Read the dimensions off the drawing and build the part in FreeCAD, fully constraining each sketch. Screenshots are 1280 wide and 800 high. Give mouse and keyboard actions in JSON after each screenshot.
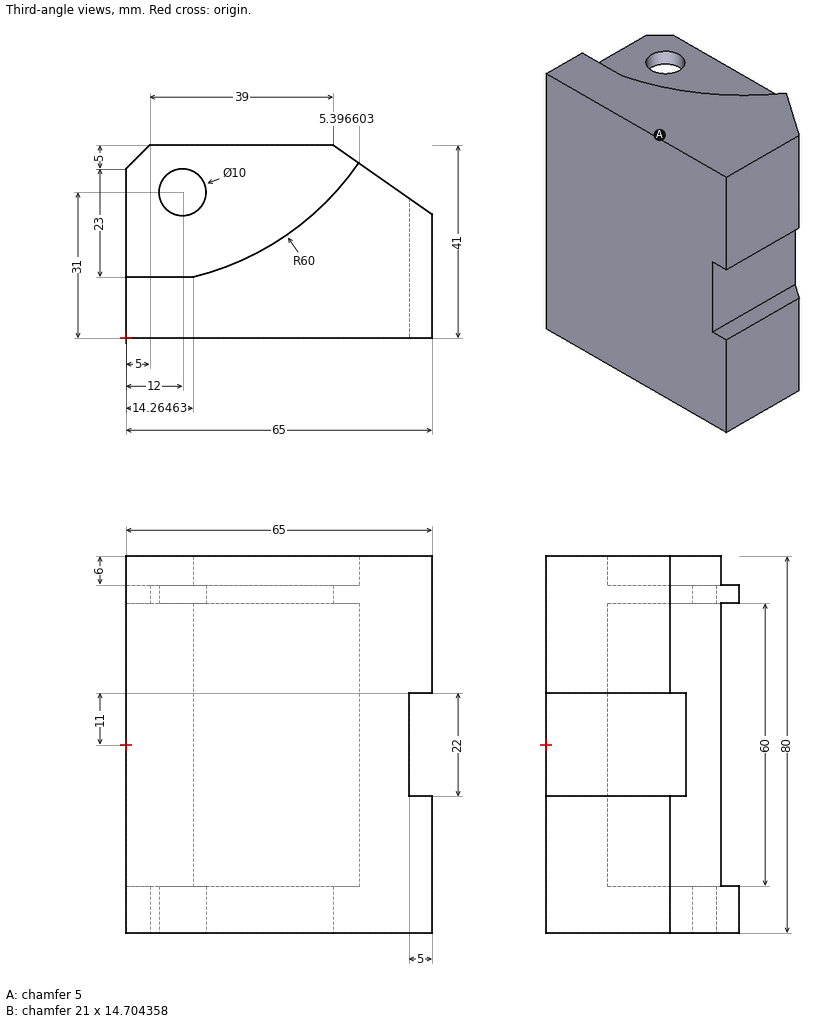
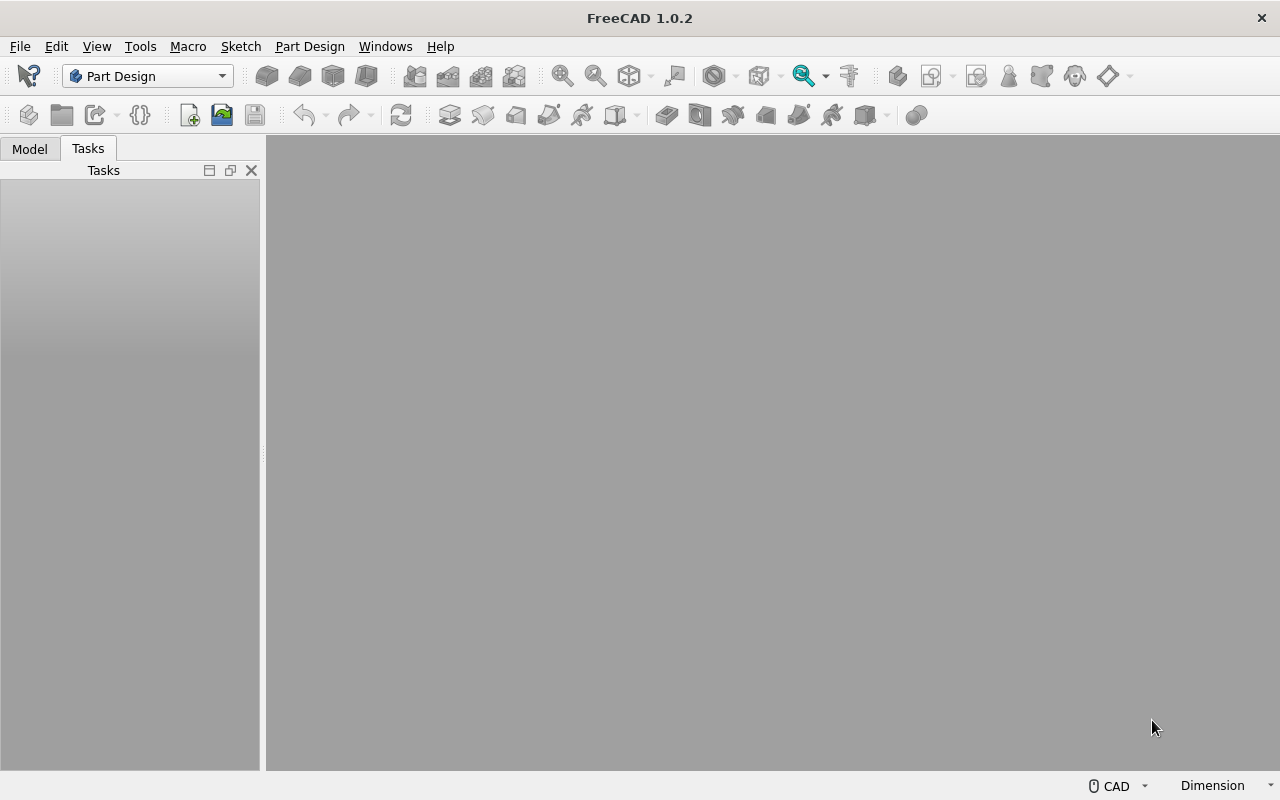
{"action": "key", "text": "ctrl+n"}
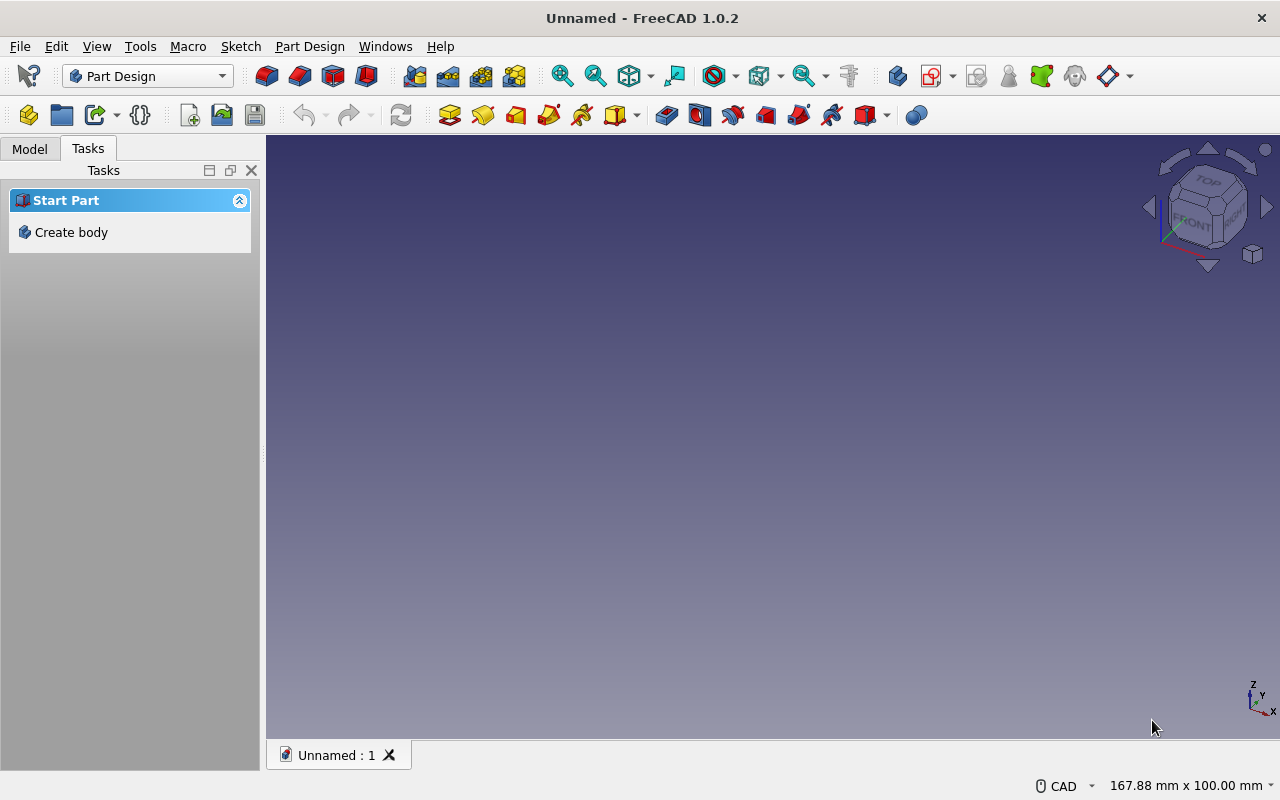
{"action": "left_click", "coordinate": [930, 76]}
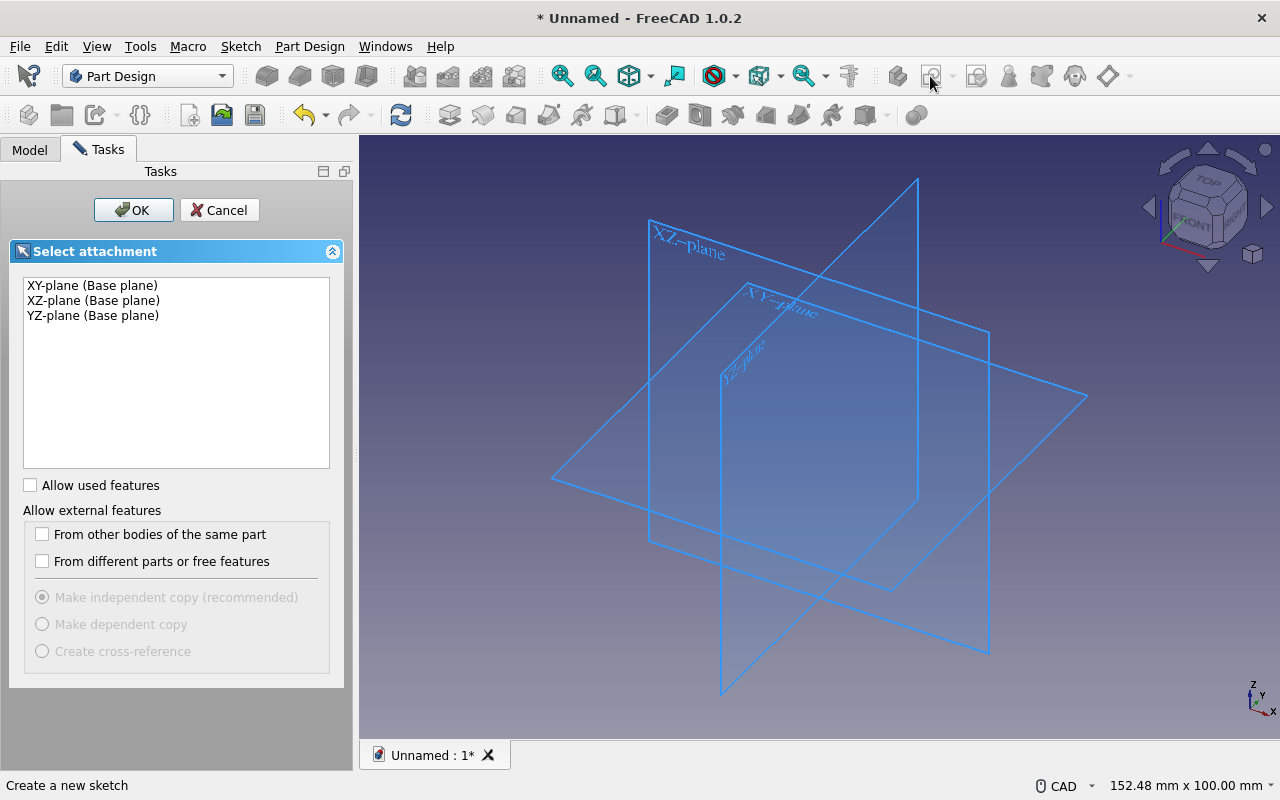
{"action": "left_click", "coordinate": [84, 286]}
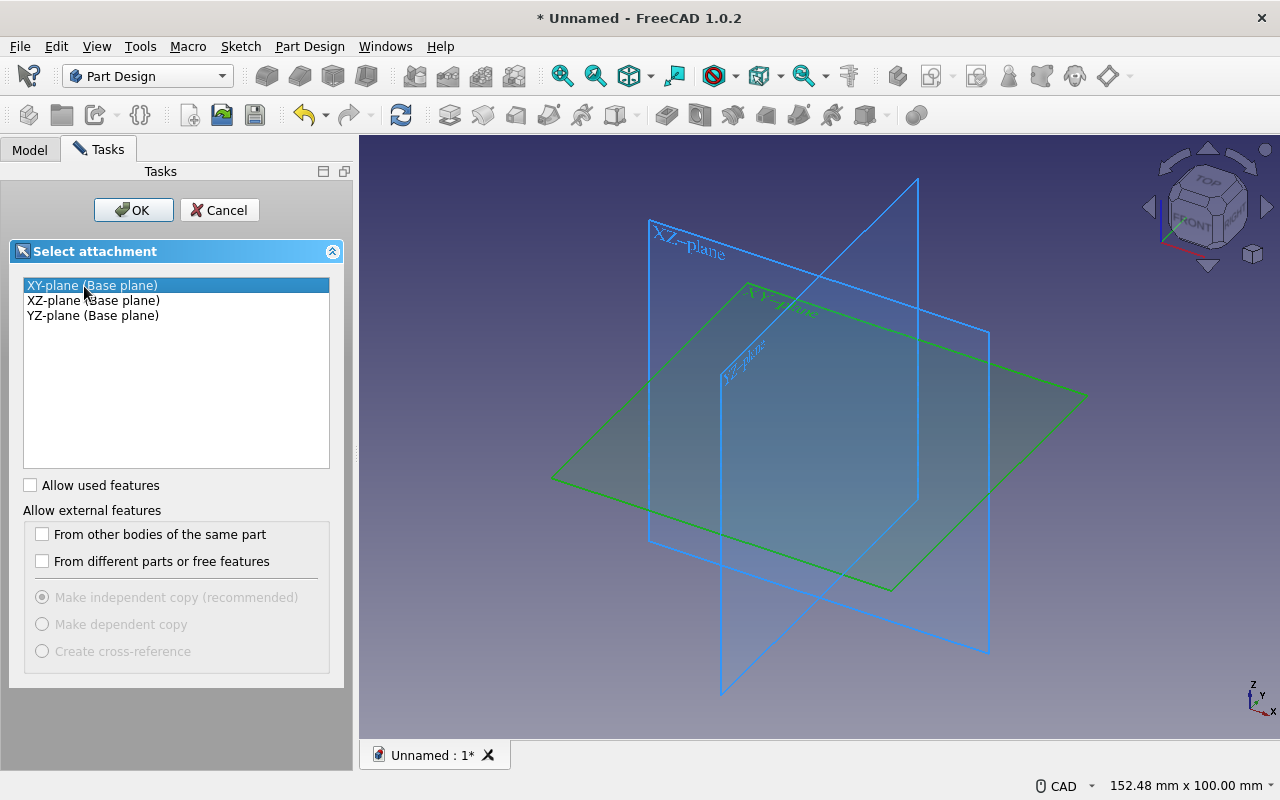
{"action": "left_click", "coordinate": [134, 210]}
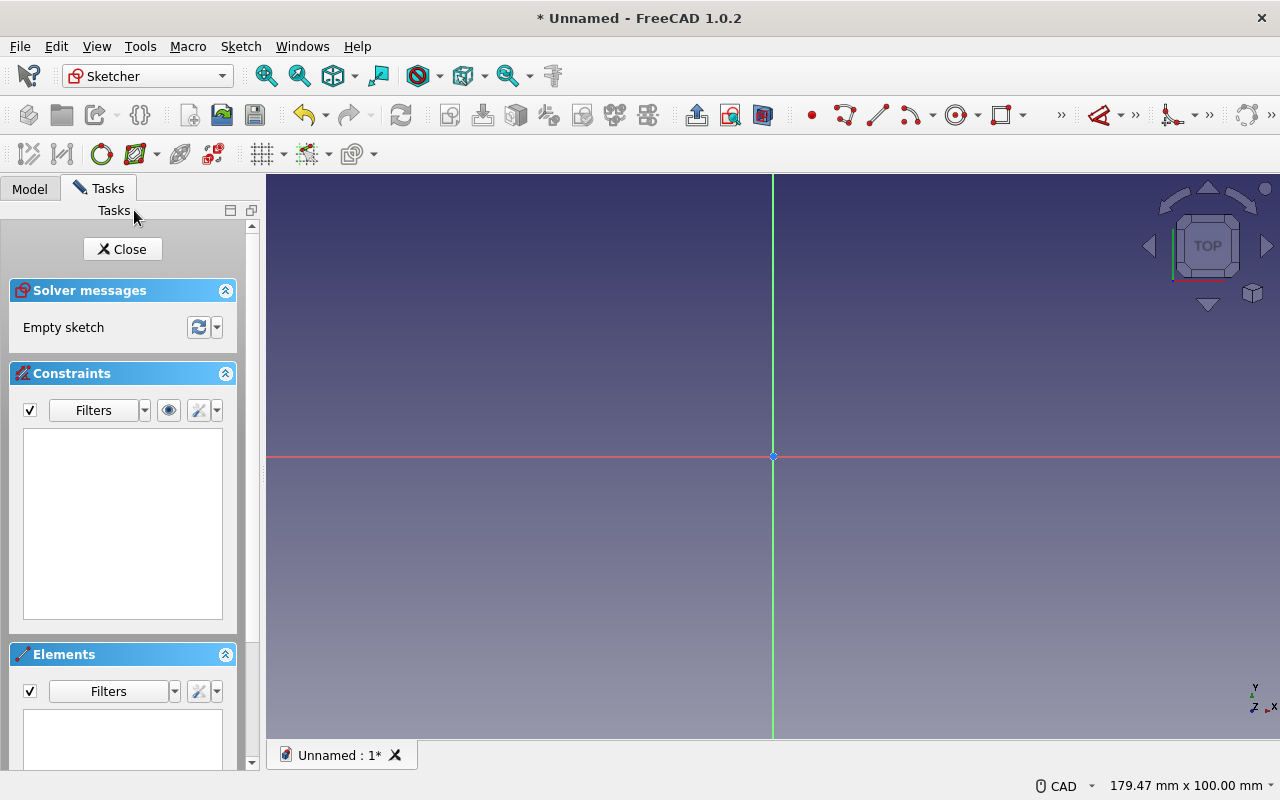
{"action": "scroll", "coordinate": [294, 711], "scroll_direction": "down", "scroll_amount": 1}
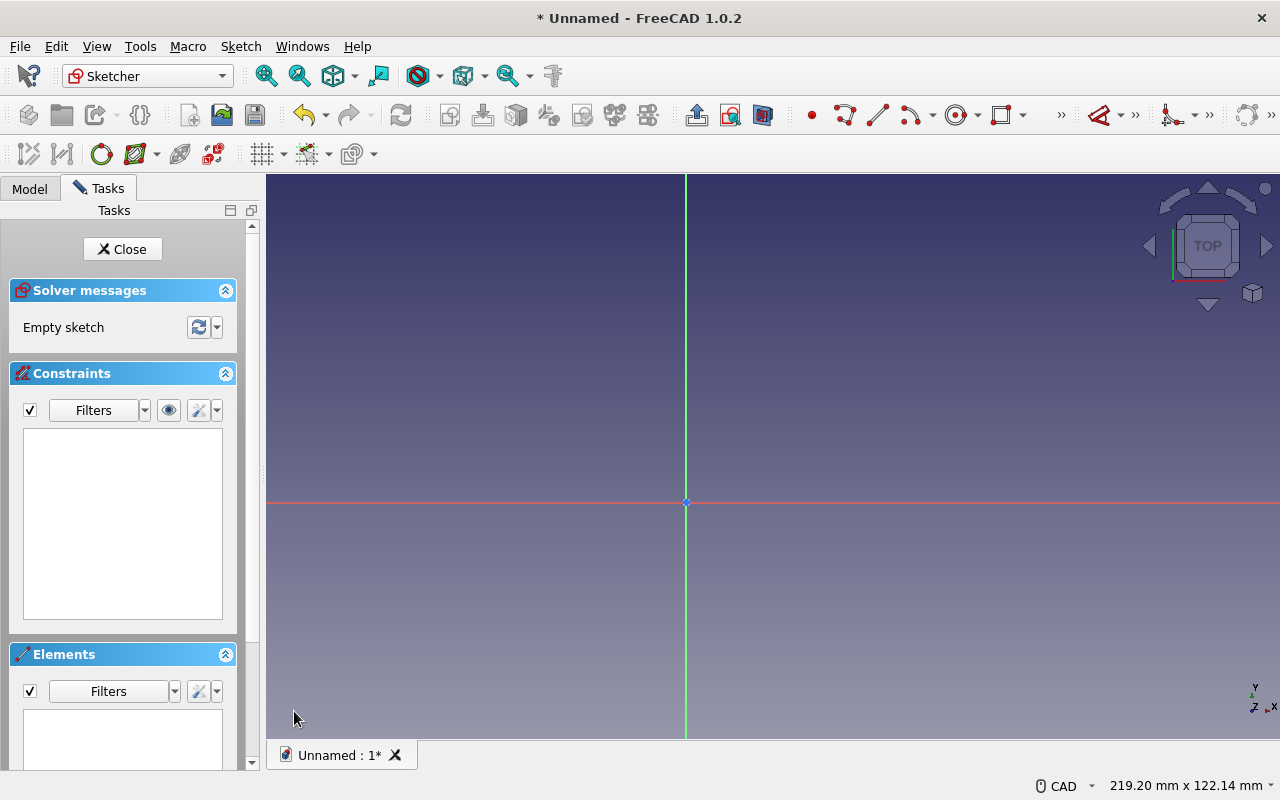
{"action": "scroll", "coordinate": [997, 349], "scroll_direction": "up", "scroll_amount": 3}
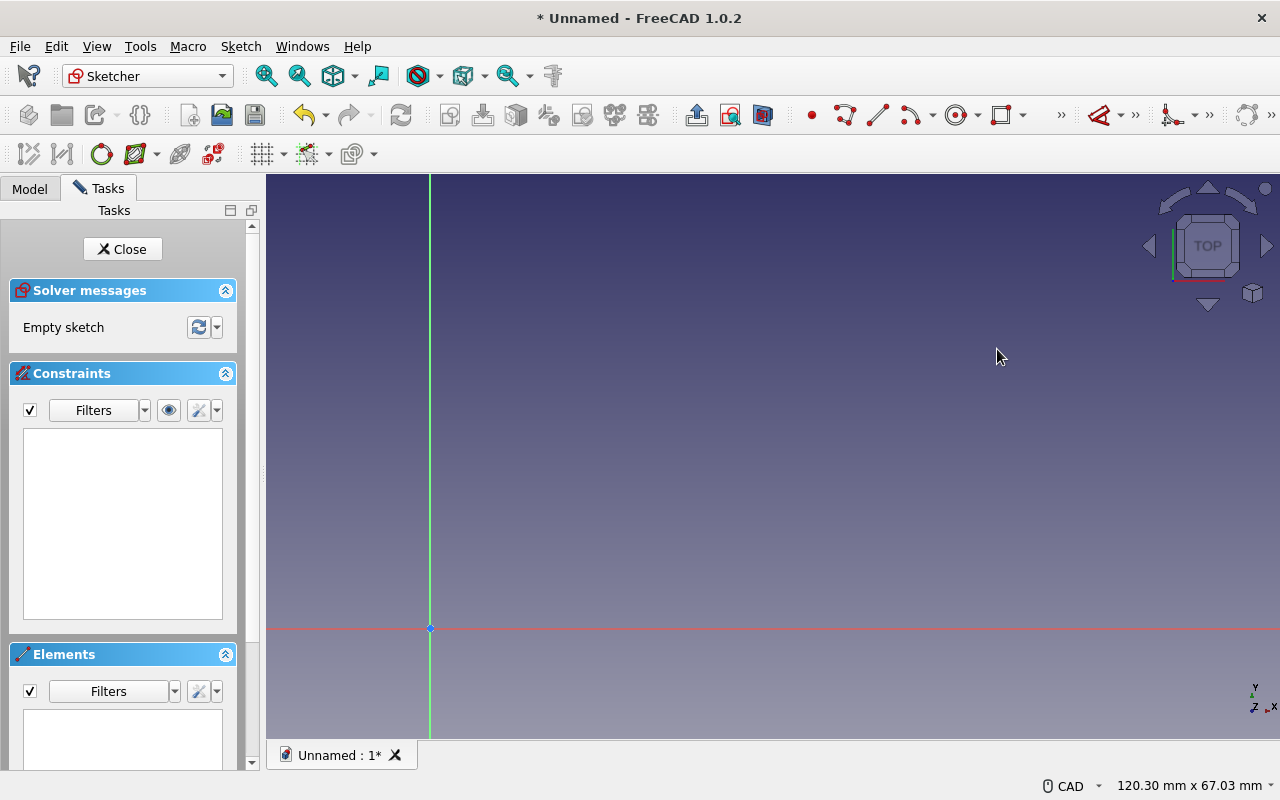
{"action": "key", "text": "g r"}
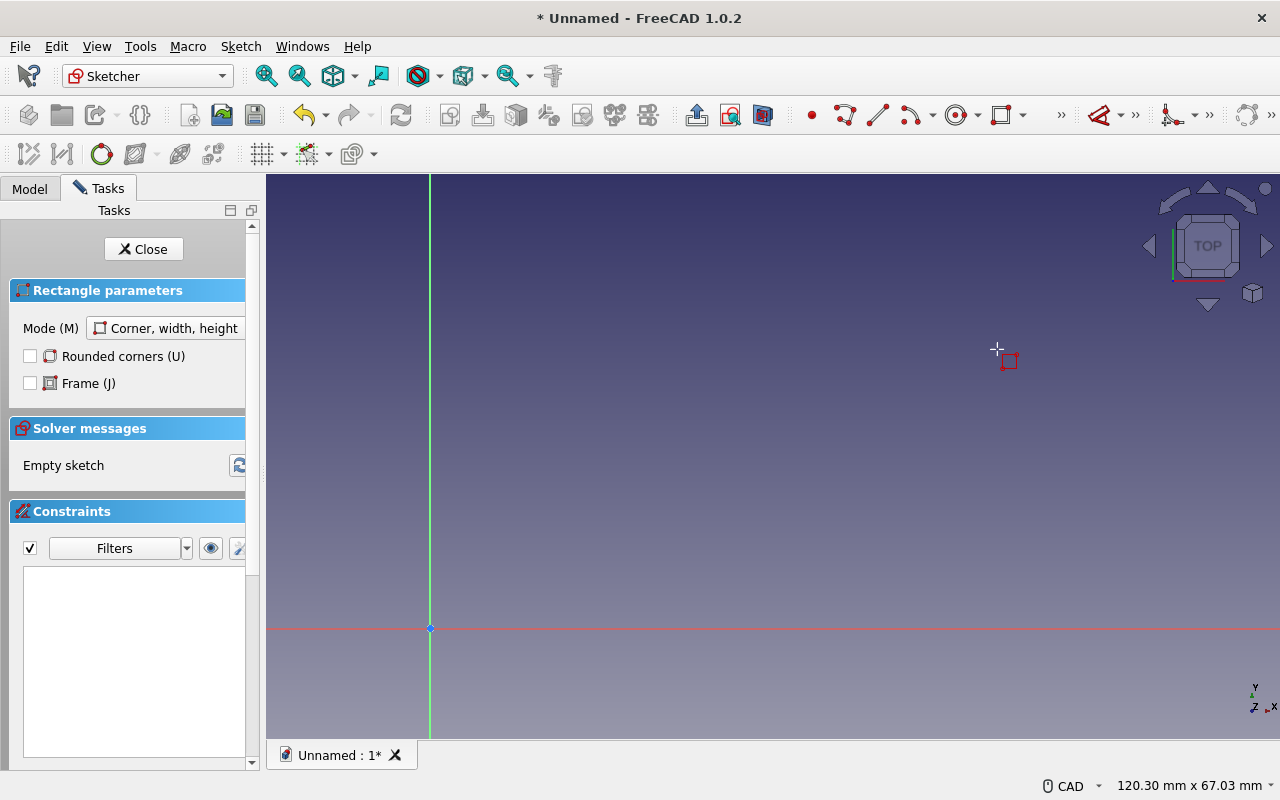
{"action": "left_click", "coordinate": [430, 629]}
{"action": "left_click", "coordinate": [978, 283]}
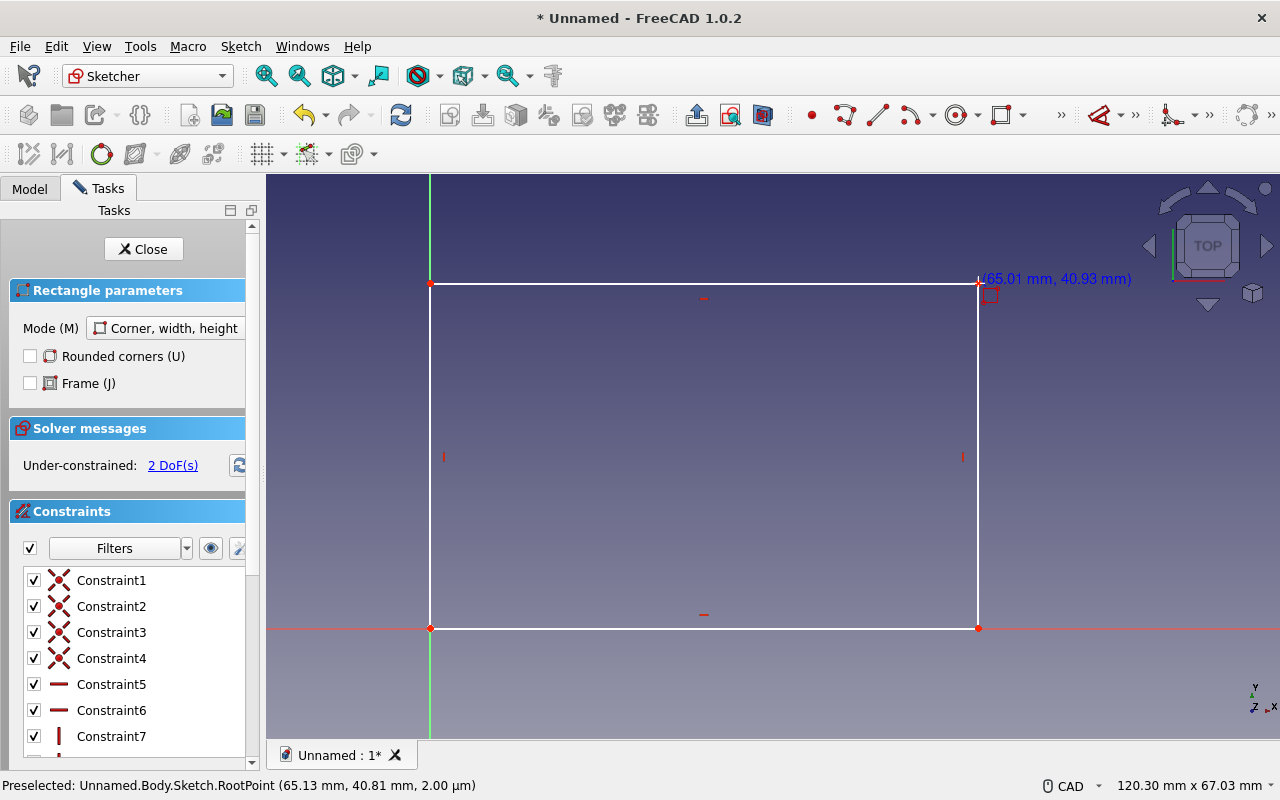
{"action": "key", "text": "g c"}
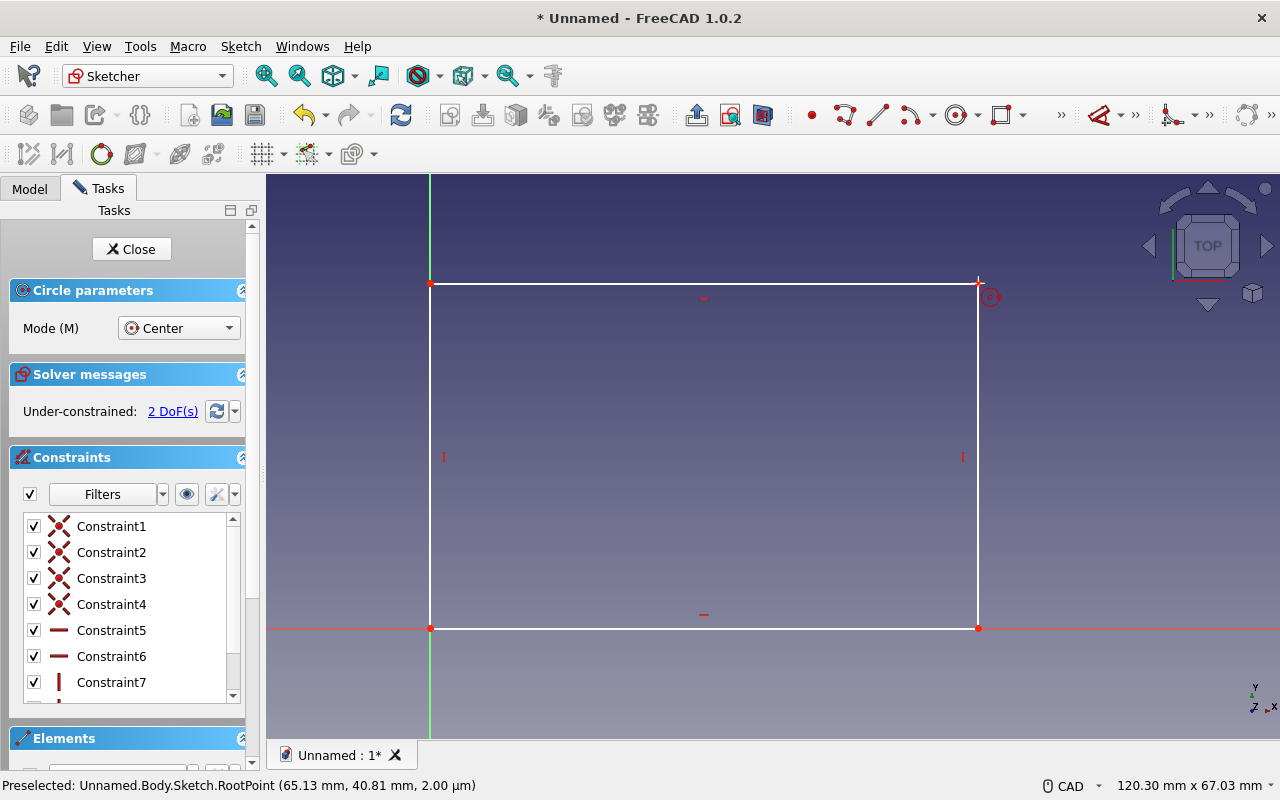
{"action": "left_click", "coordinate": [531, 368]}
{"action": "left_click", "coordinate": [561, 338]}
{"action": "key", "text": "Escape"}